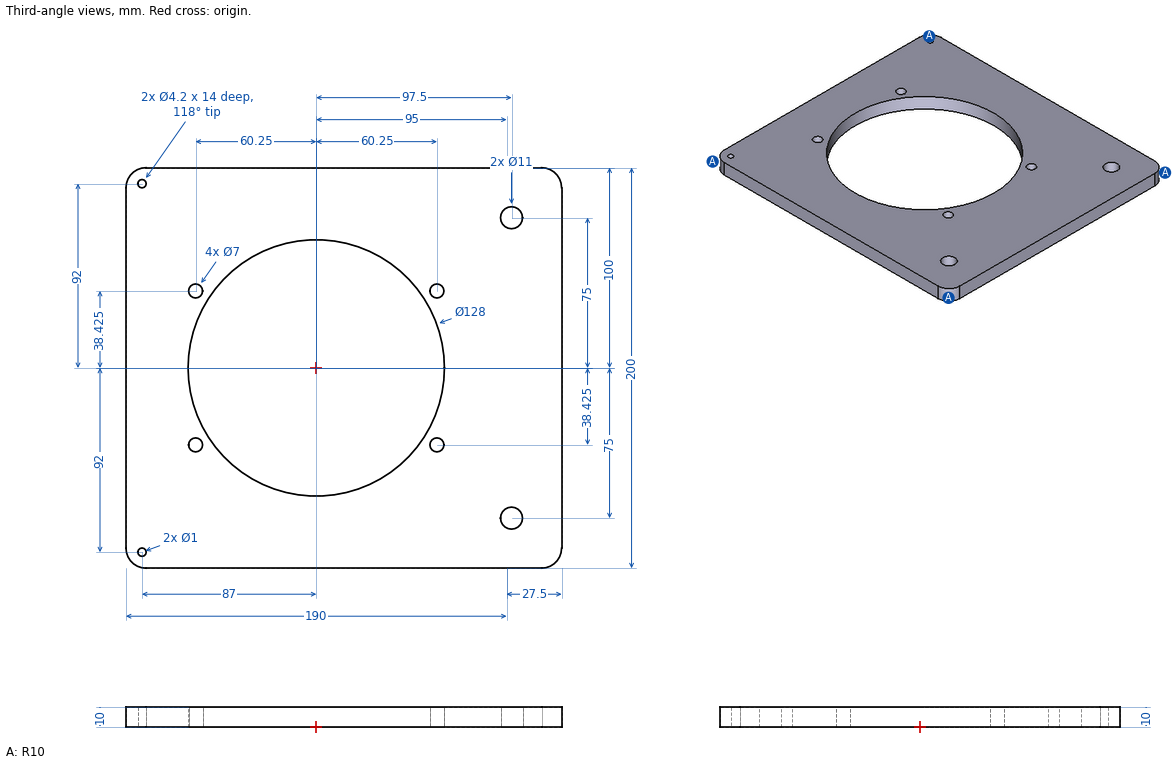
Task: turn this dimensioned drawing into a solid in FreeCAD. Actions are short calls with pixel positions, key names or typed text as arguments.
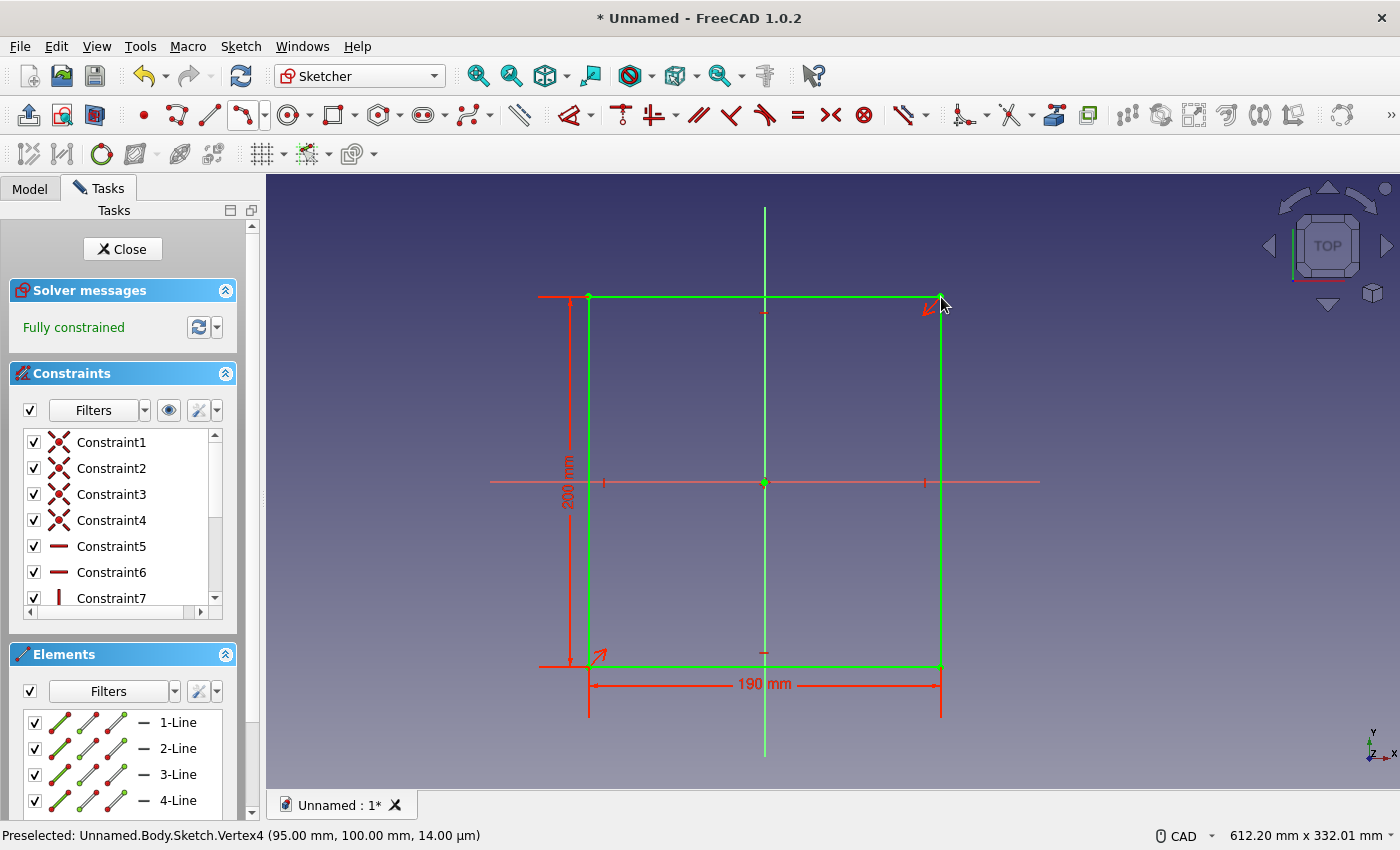
click(123, 249)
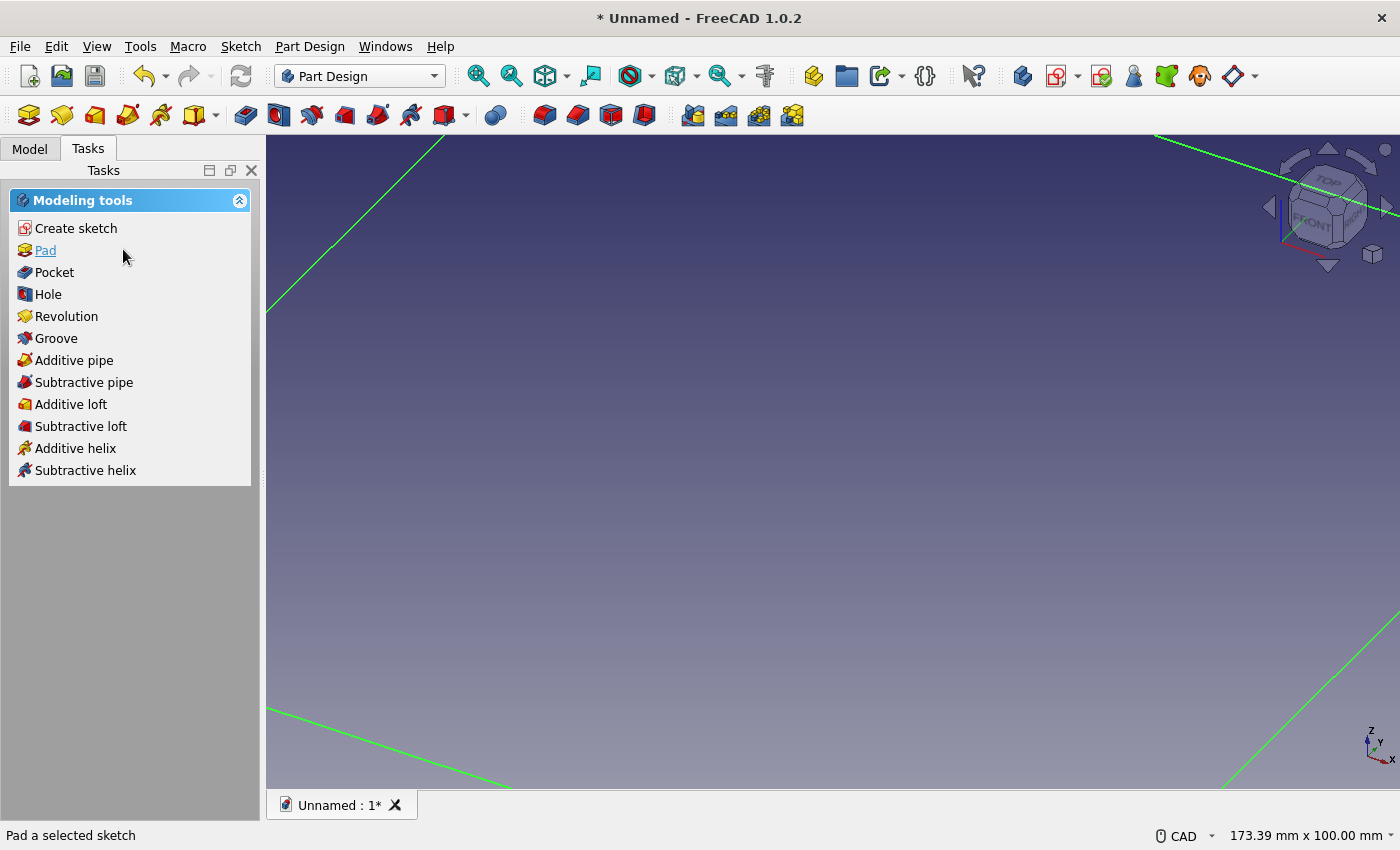
click(29, 116)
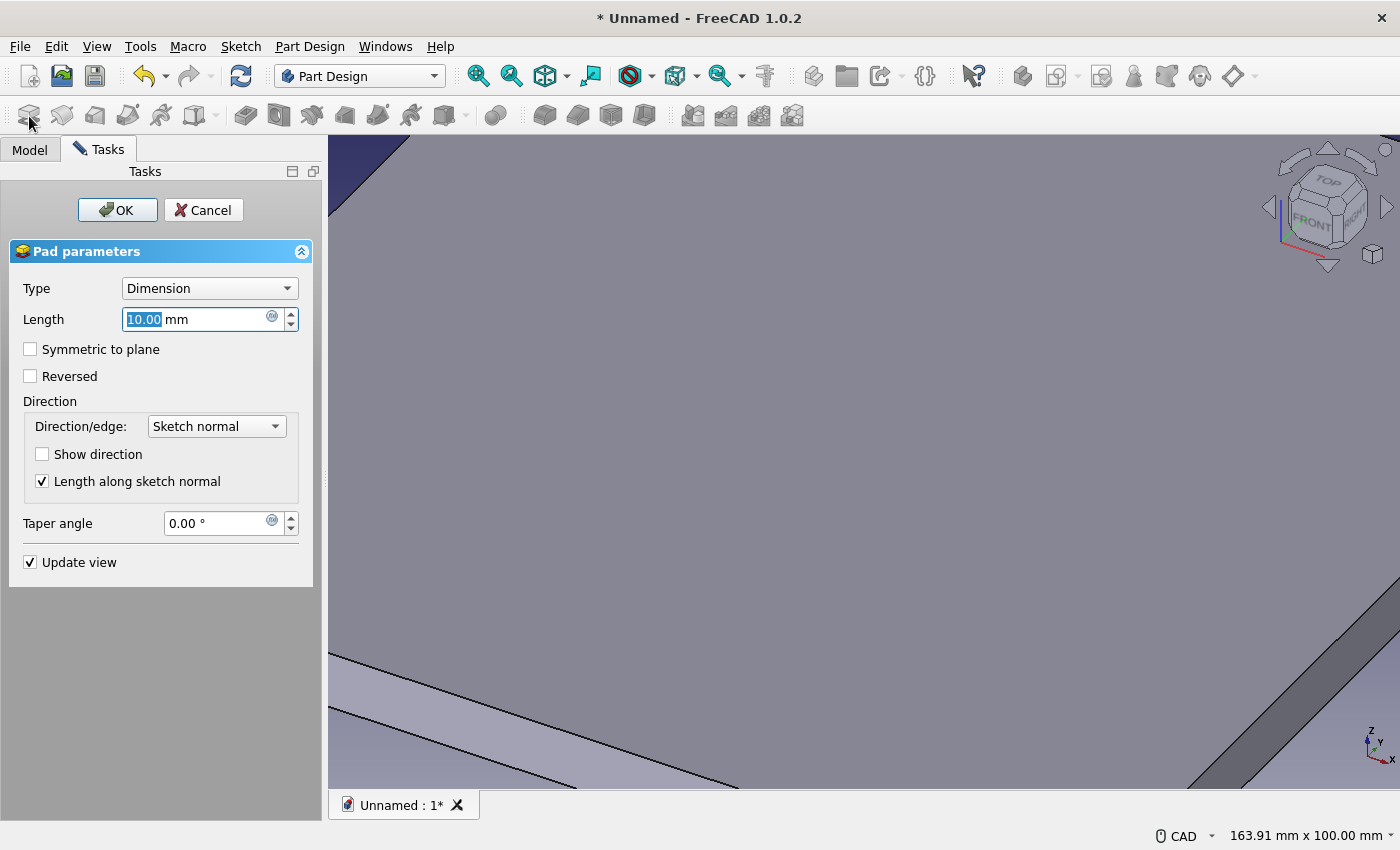
text(10)
key(Tab)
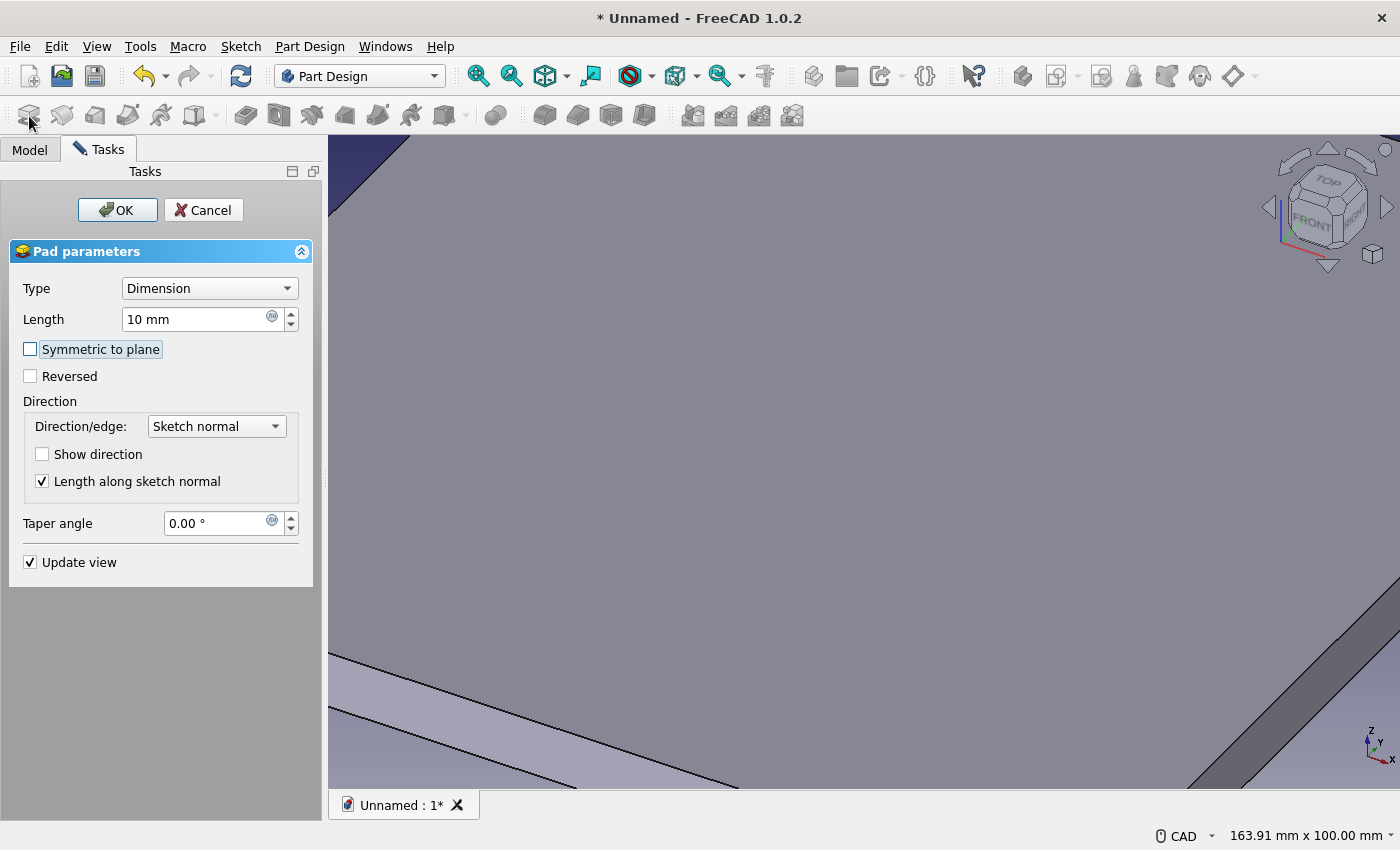
click(118, 210)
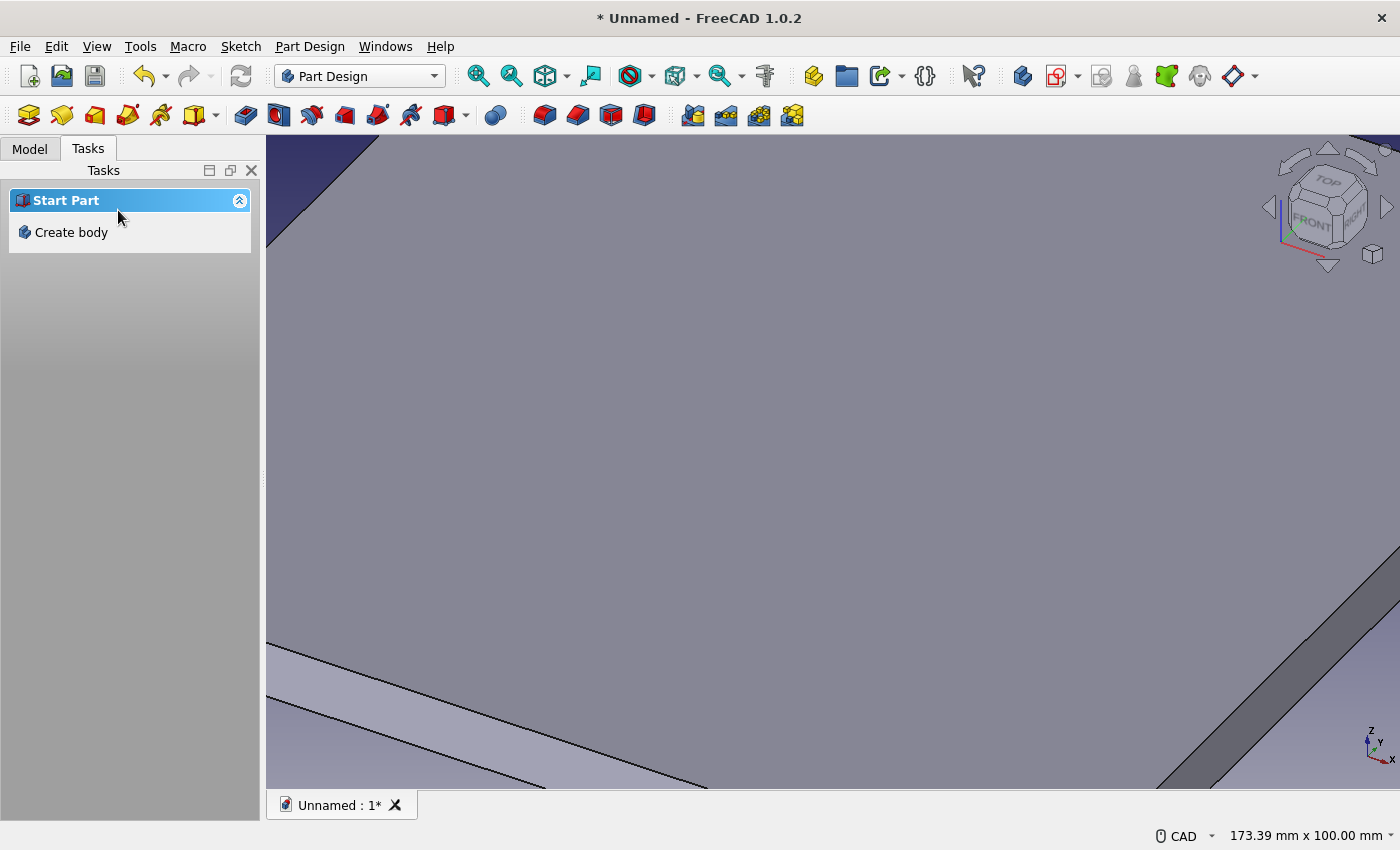
key(v)
key(f)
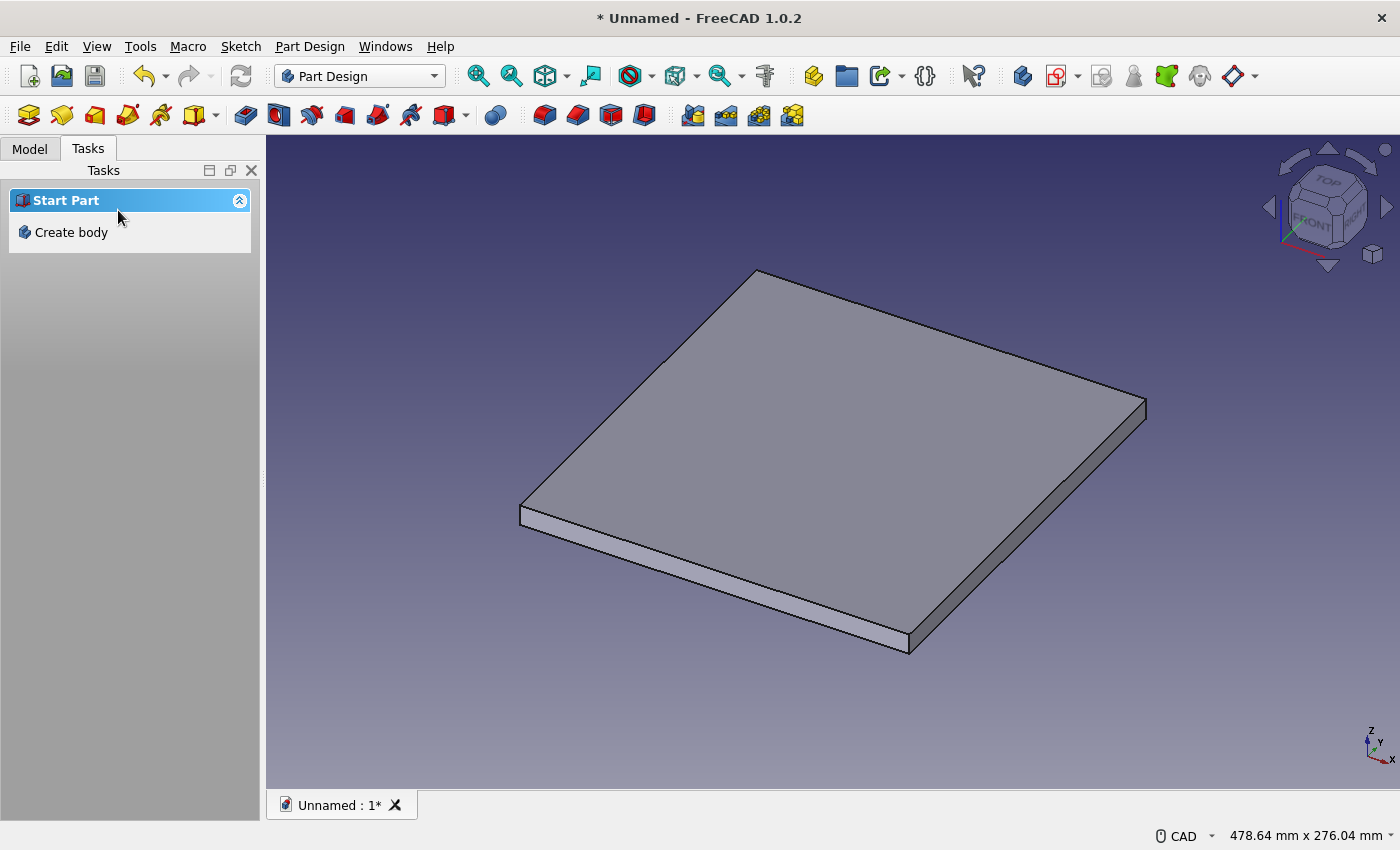
click(833, 451)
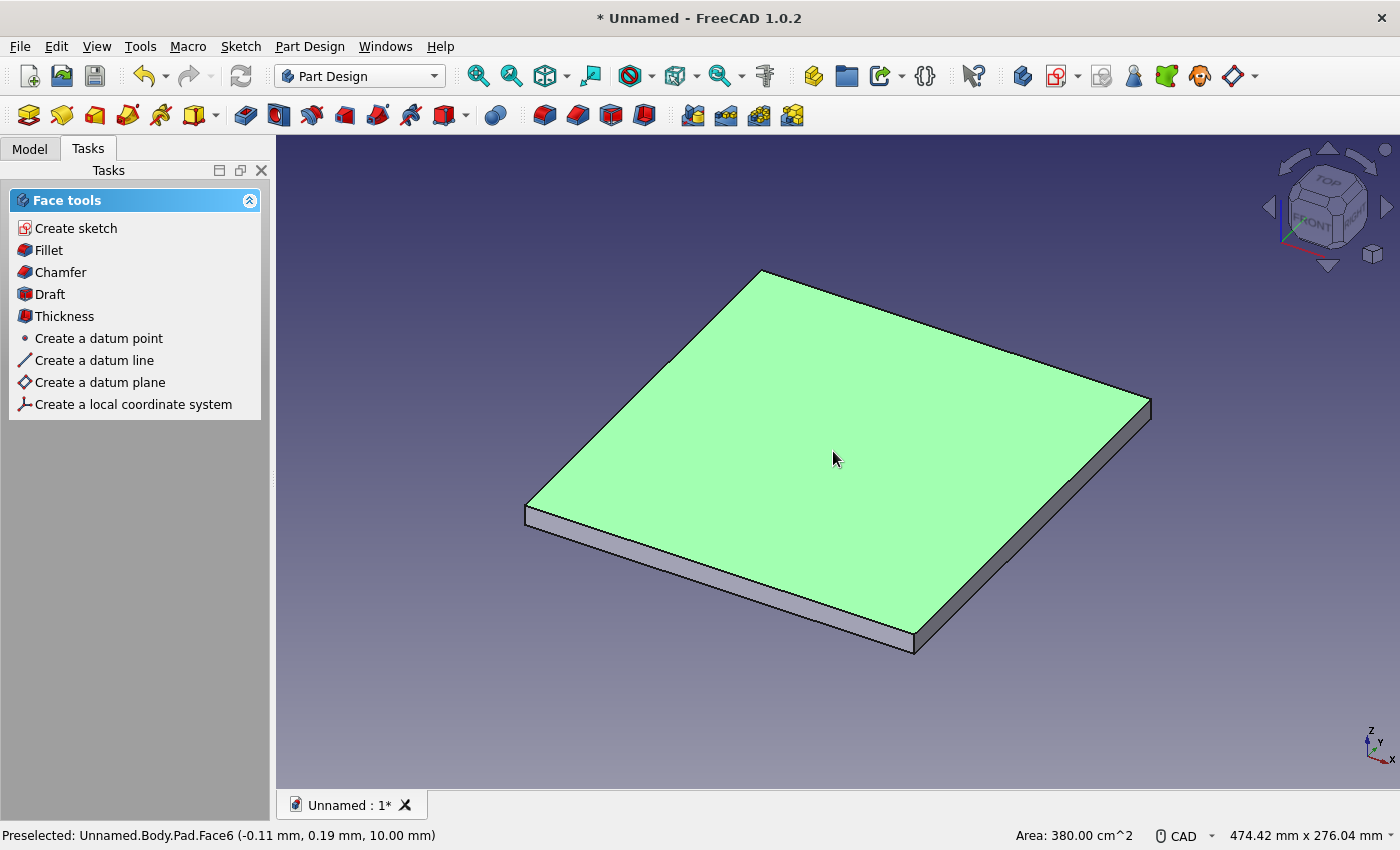
click(1056, 76)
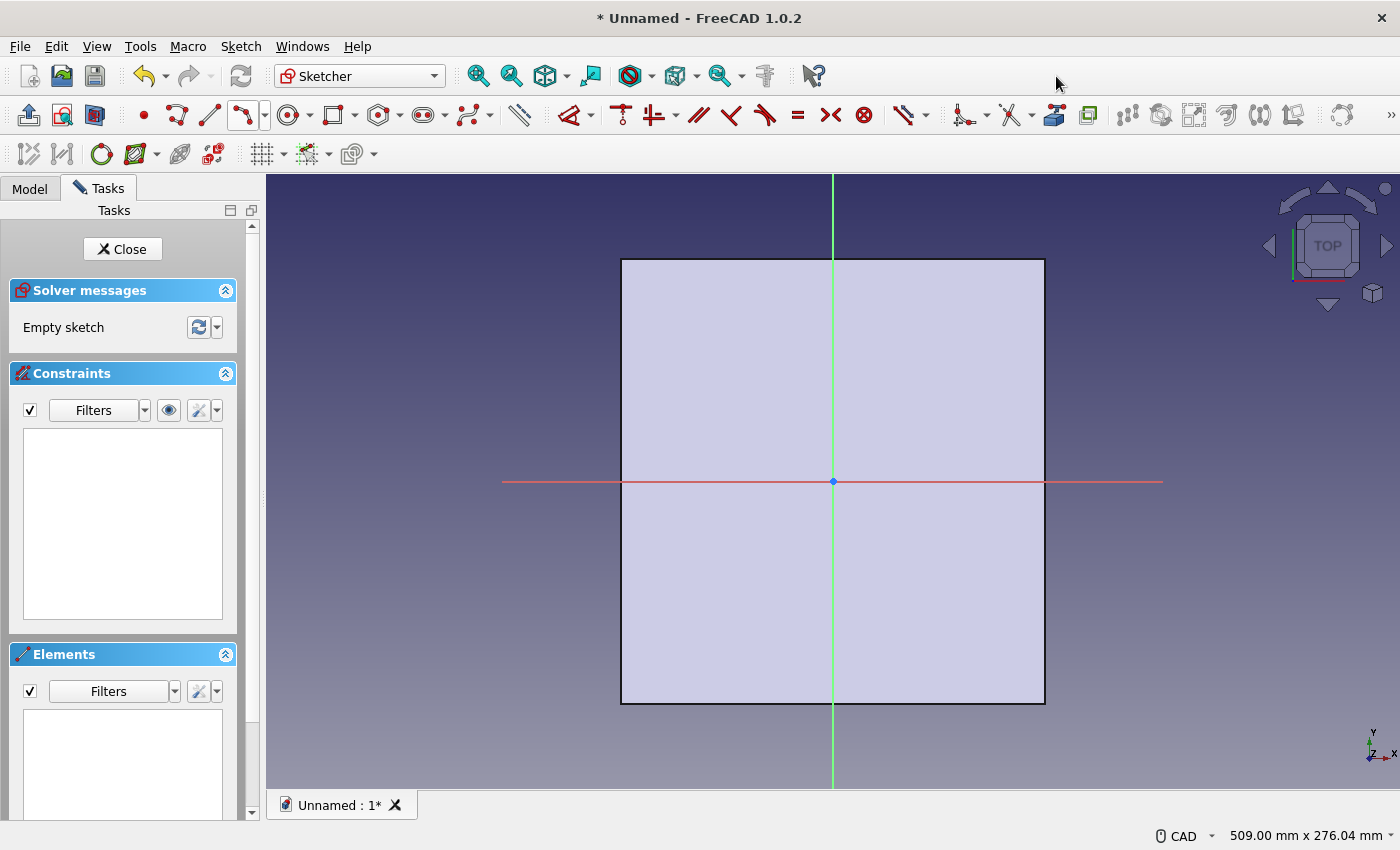
scroll(972, 482, up, 2)